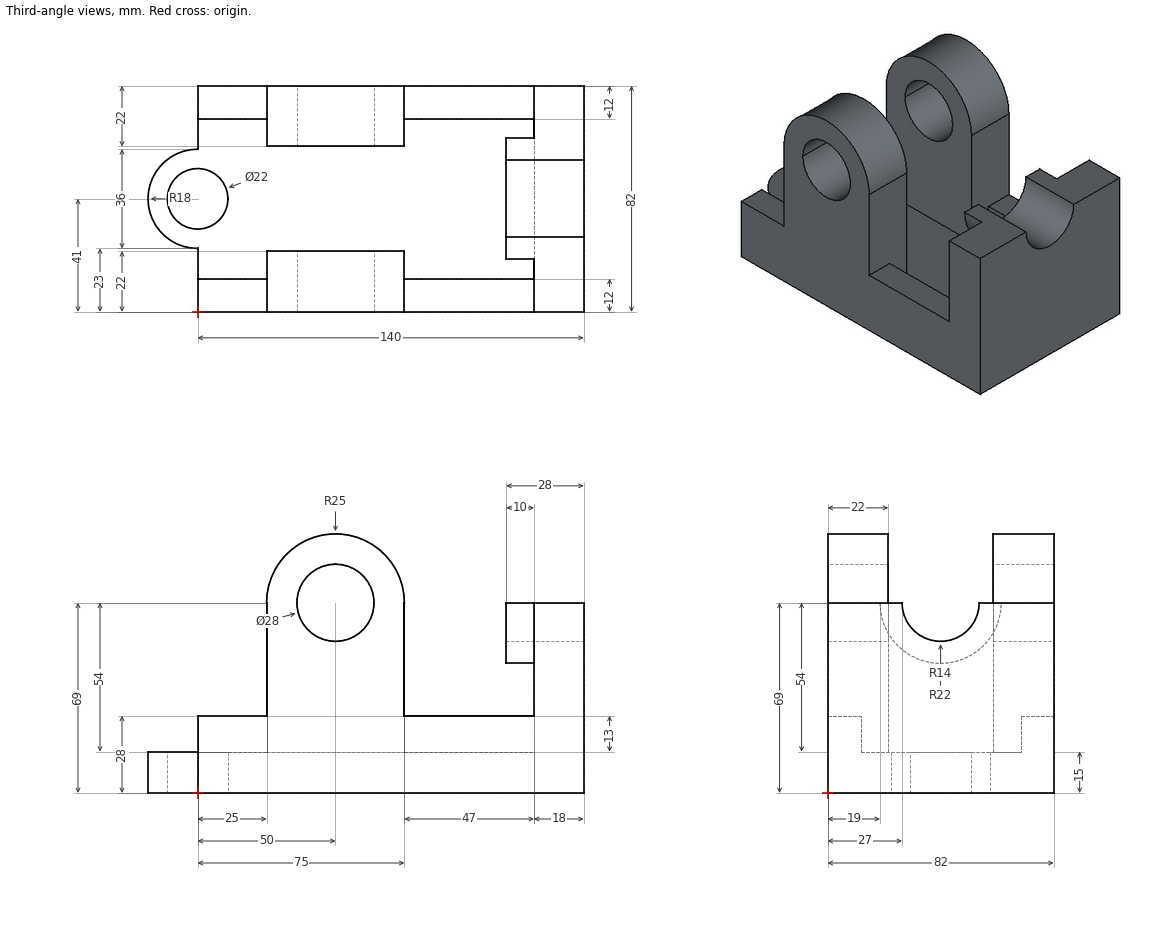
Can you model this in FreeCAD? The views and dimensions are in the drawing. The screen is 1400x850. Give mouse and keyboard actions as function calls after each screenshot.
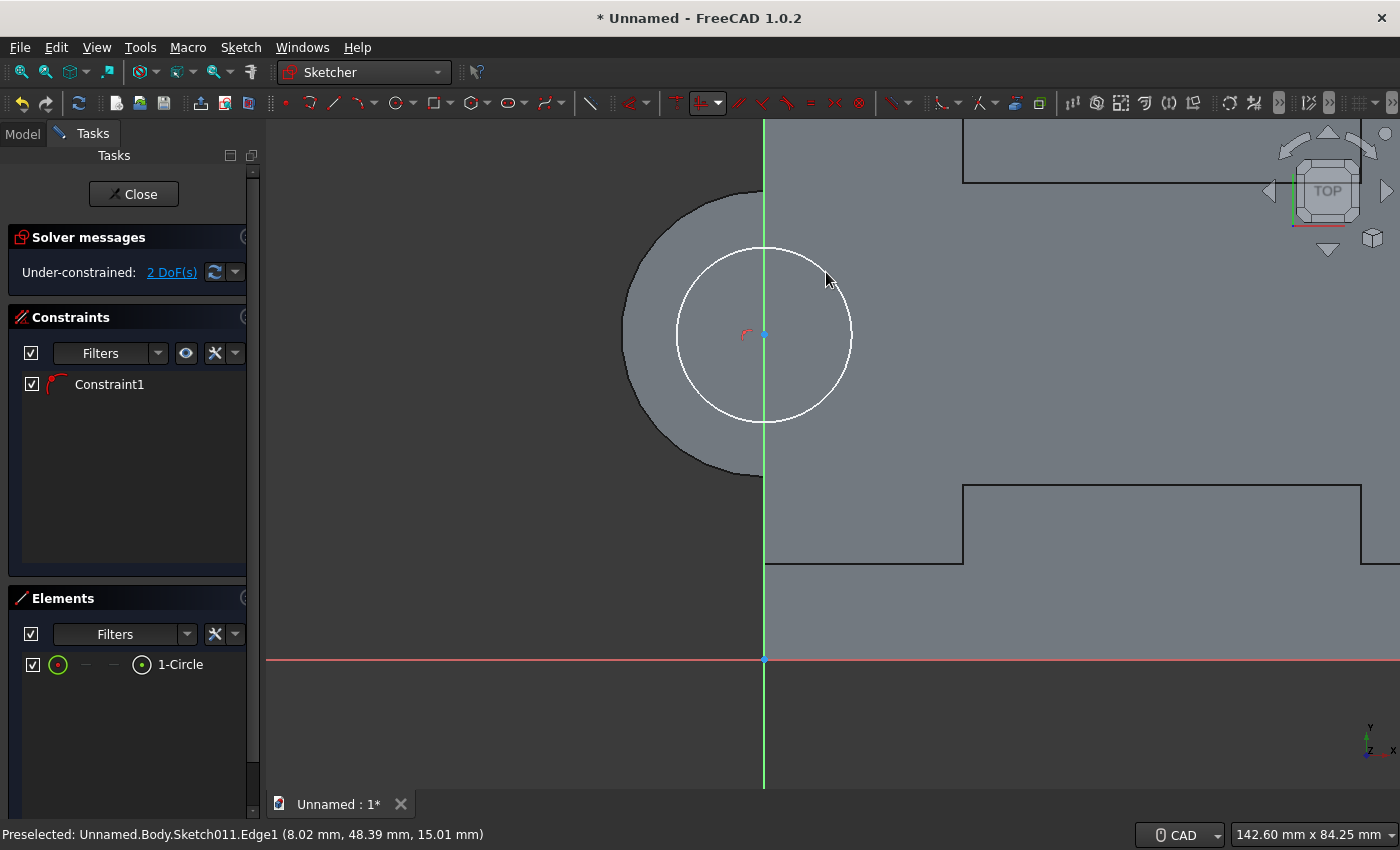
click(630, 104)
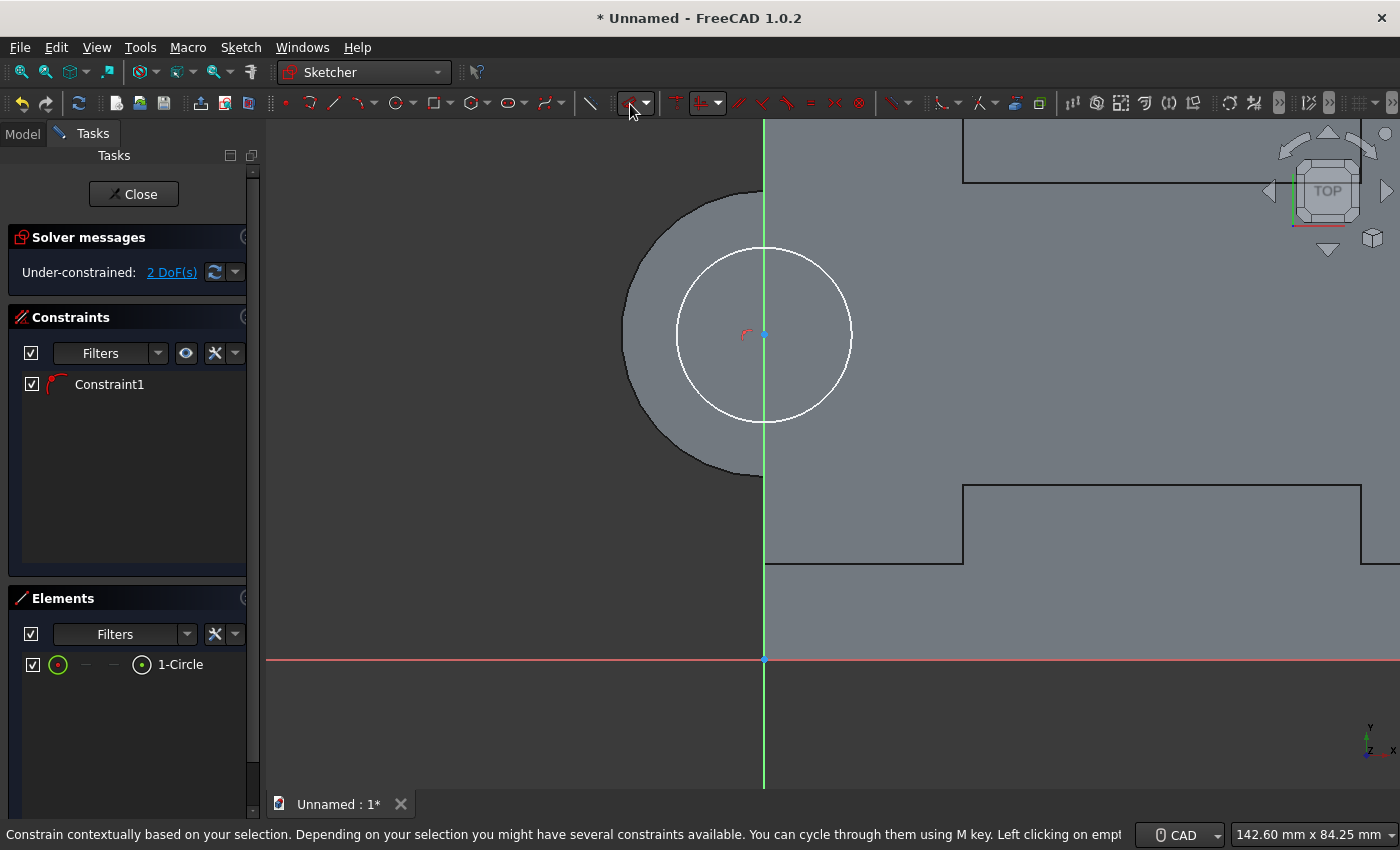
click(826, 273)
click(849, 250)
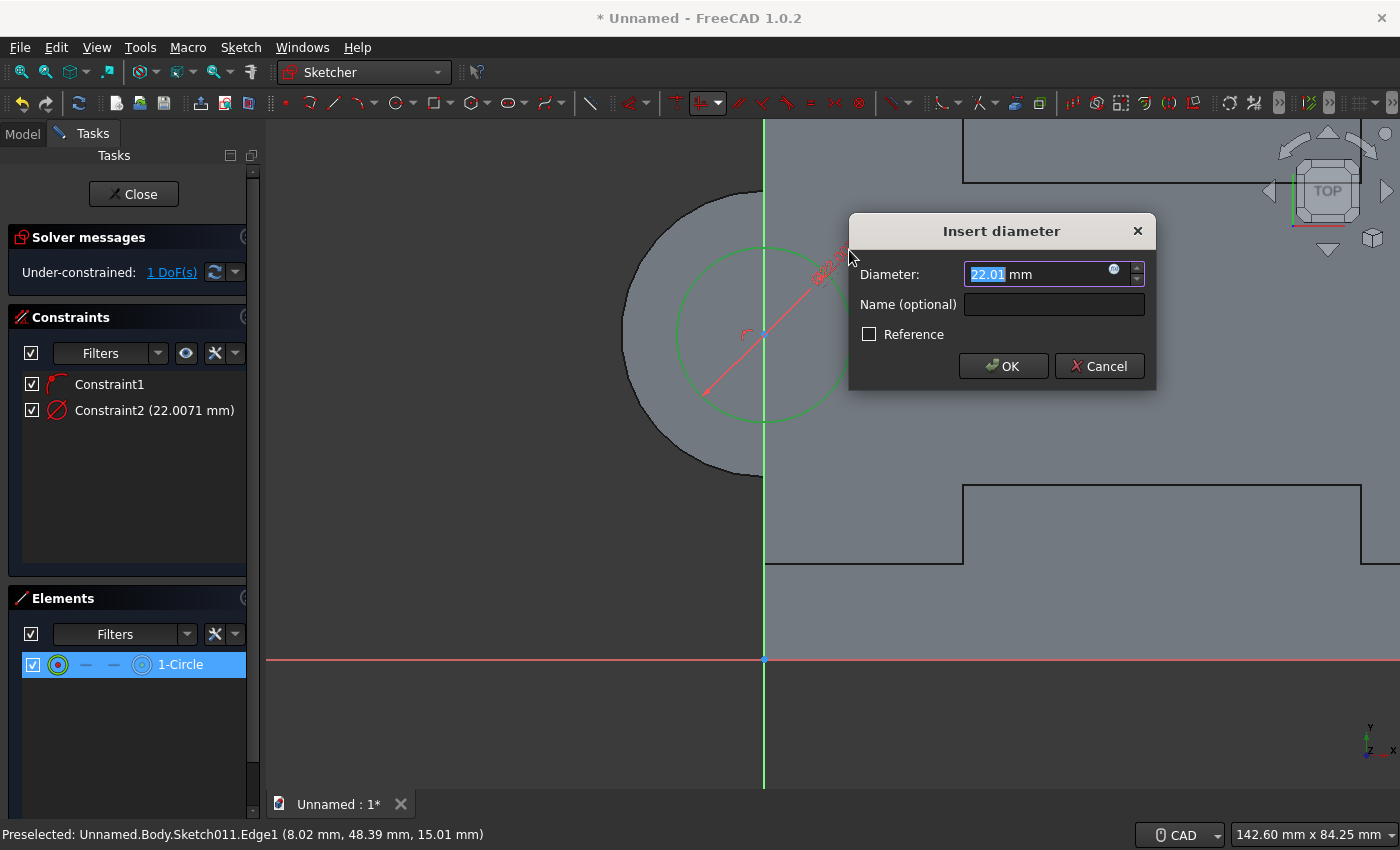
text(22)
key(Return)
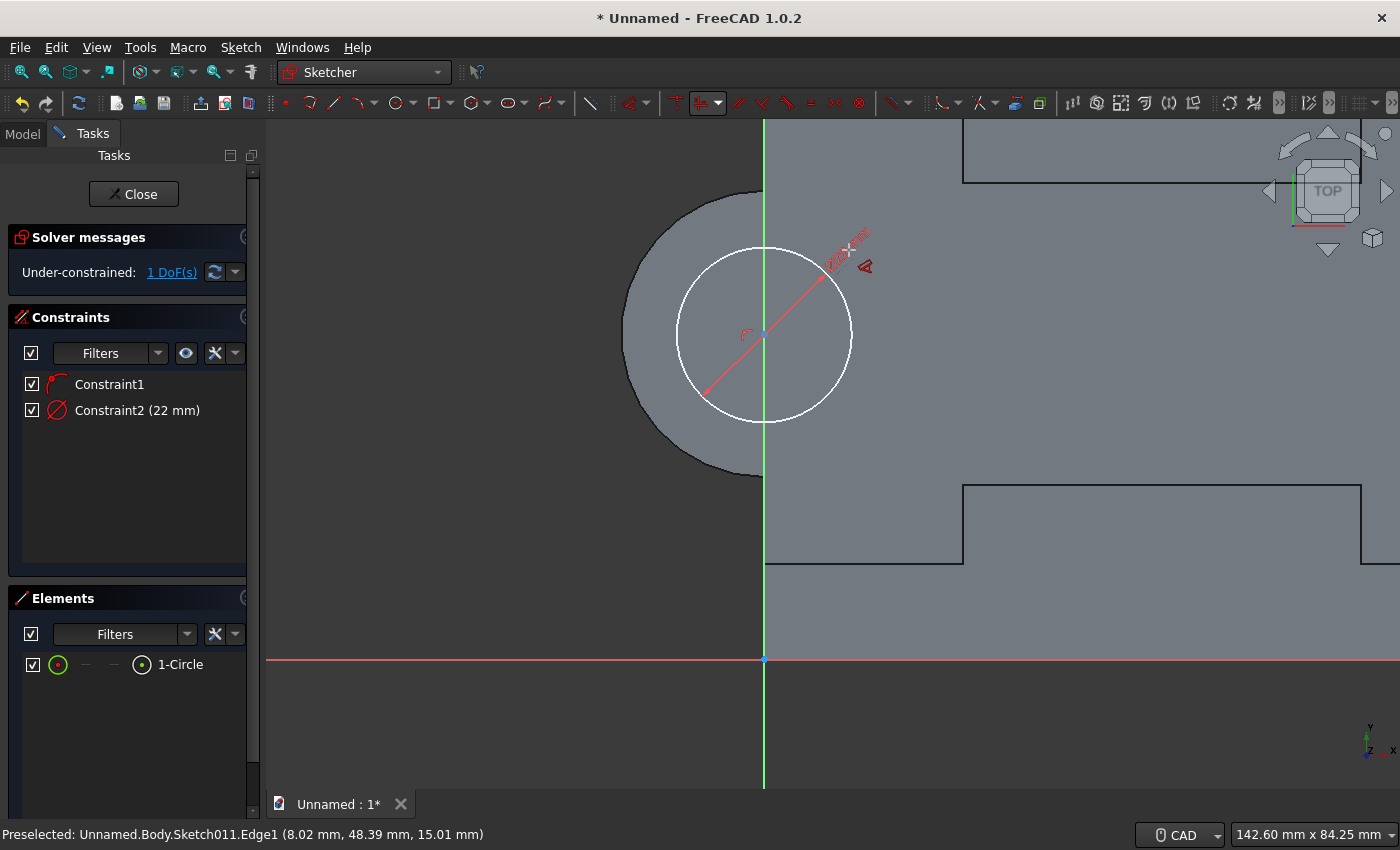
click(764, 335)
click(798, 497)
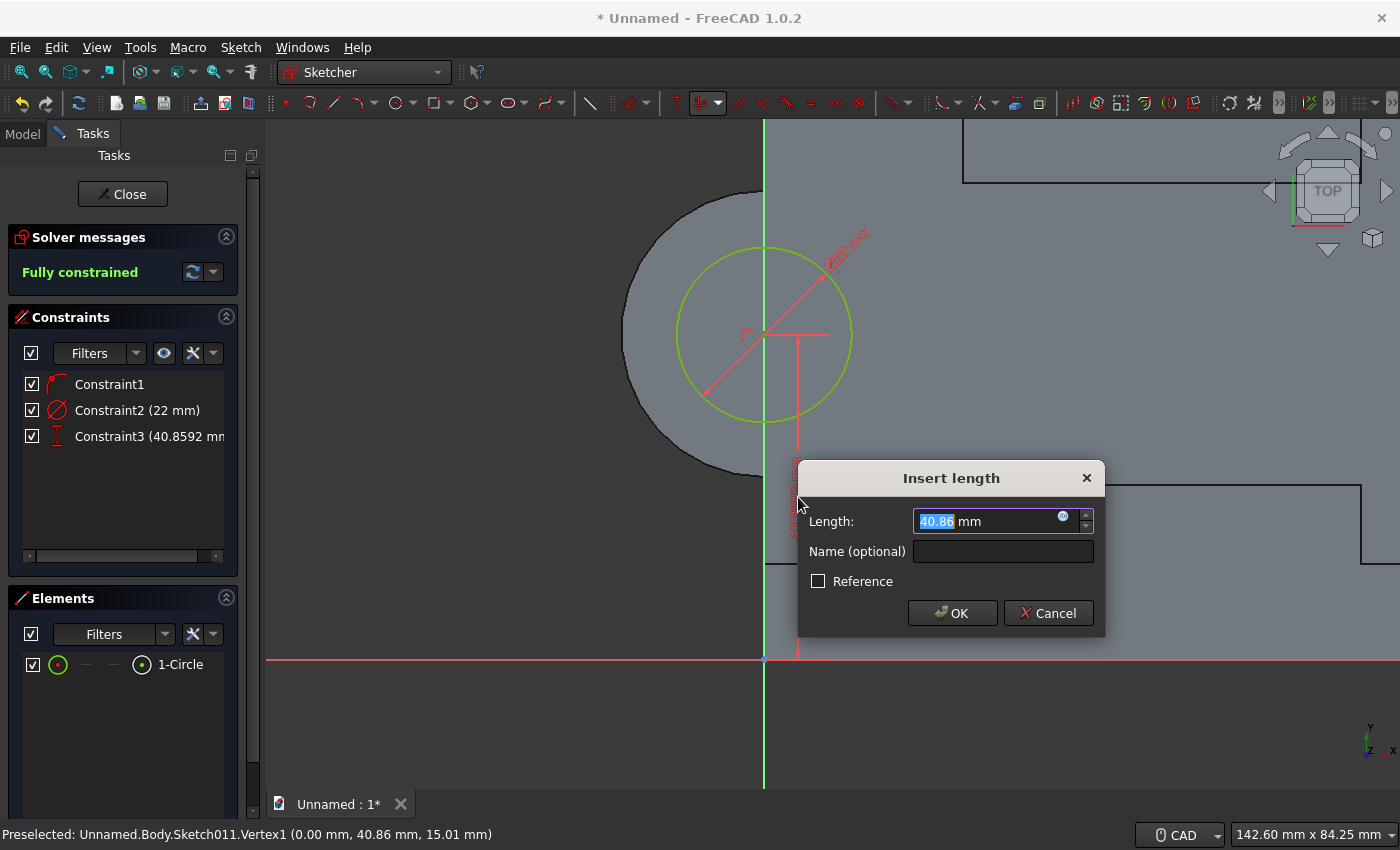
text(41)
key(Return)
key(Escape)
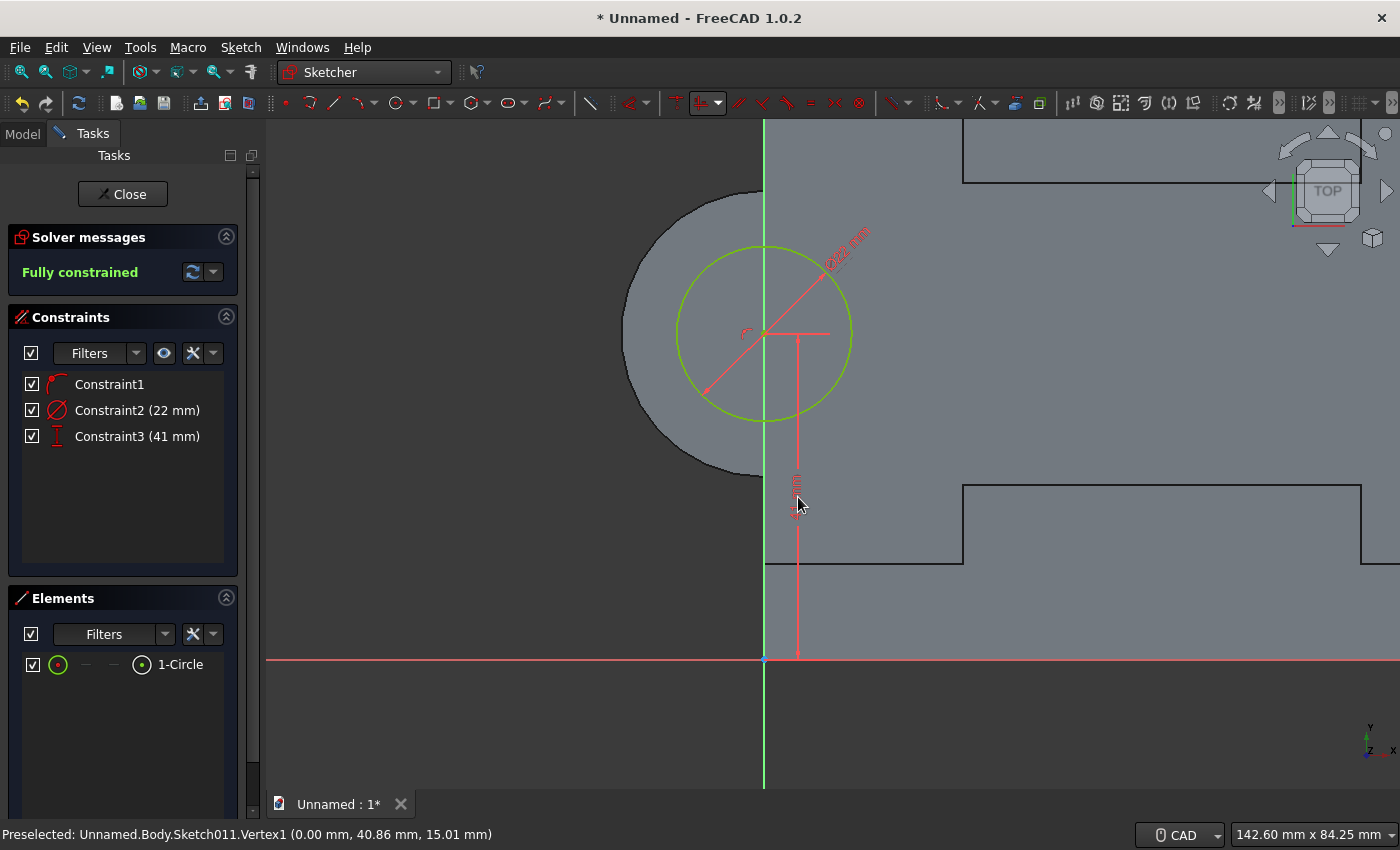
click(123, 194)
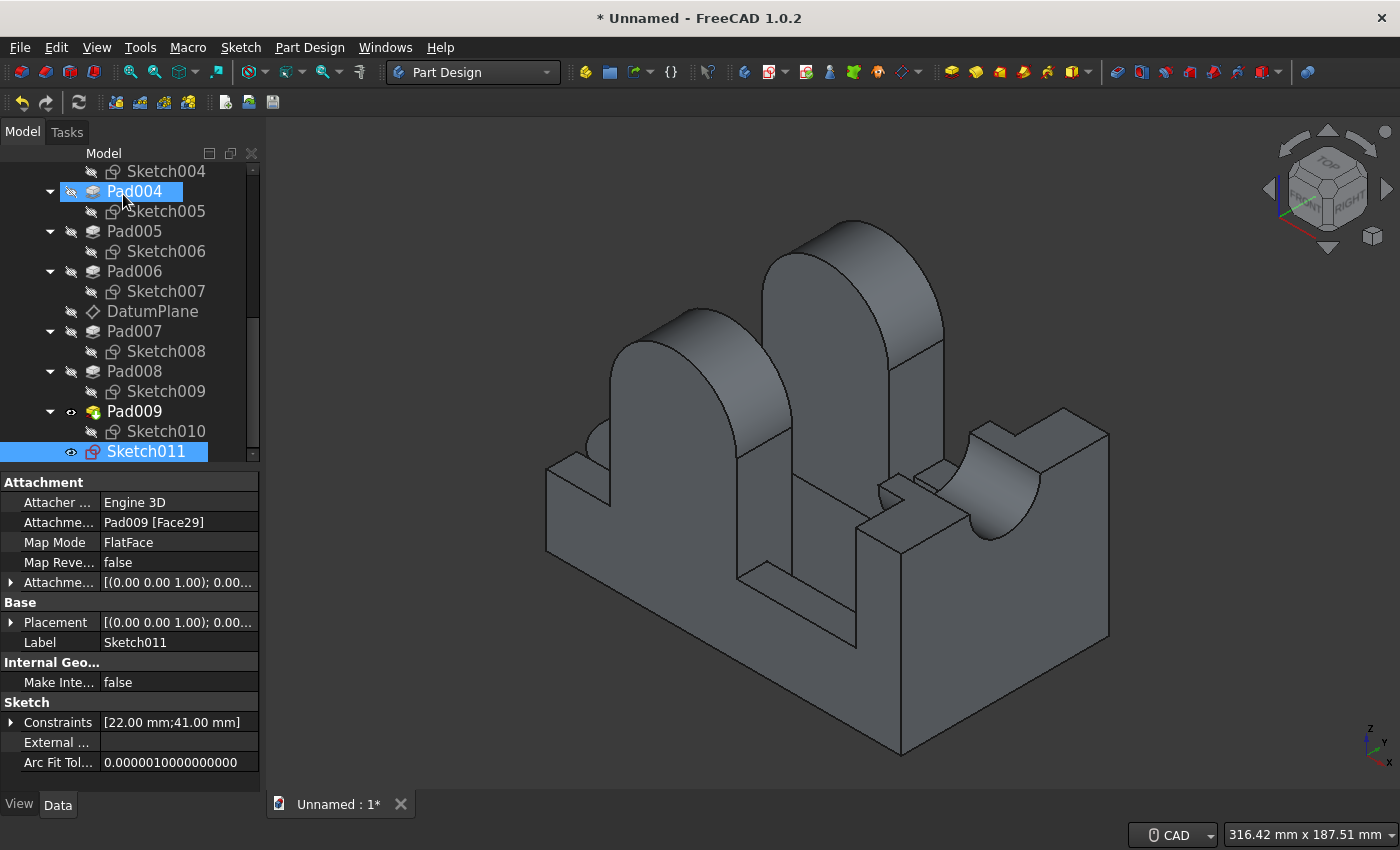
click(1118, 72)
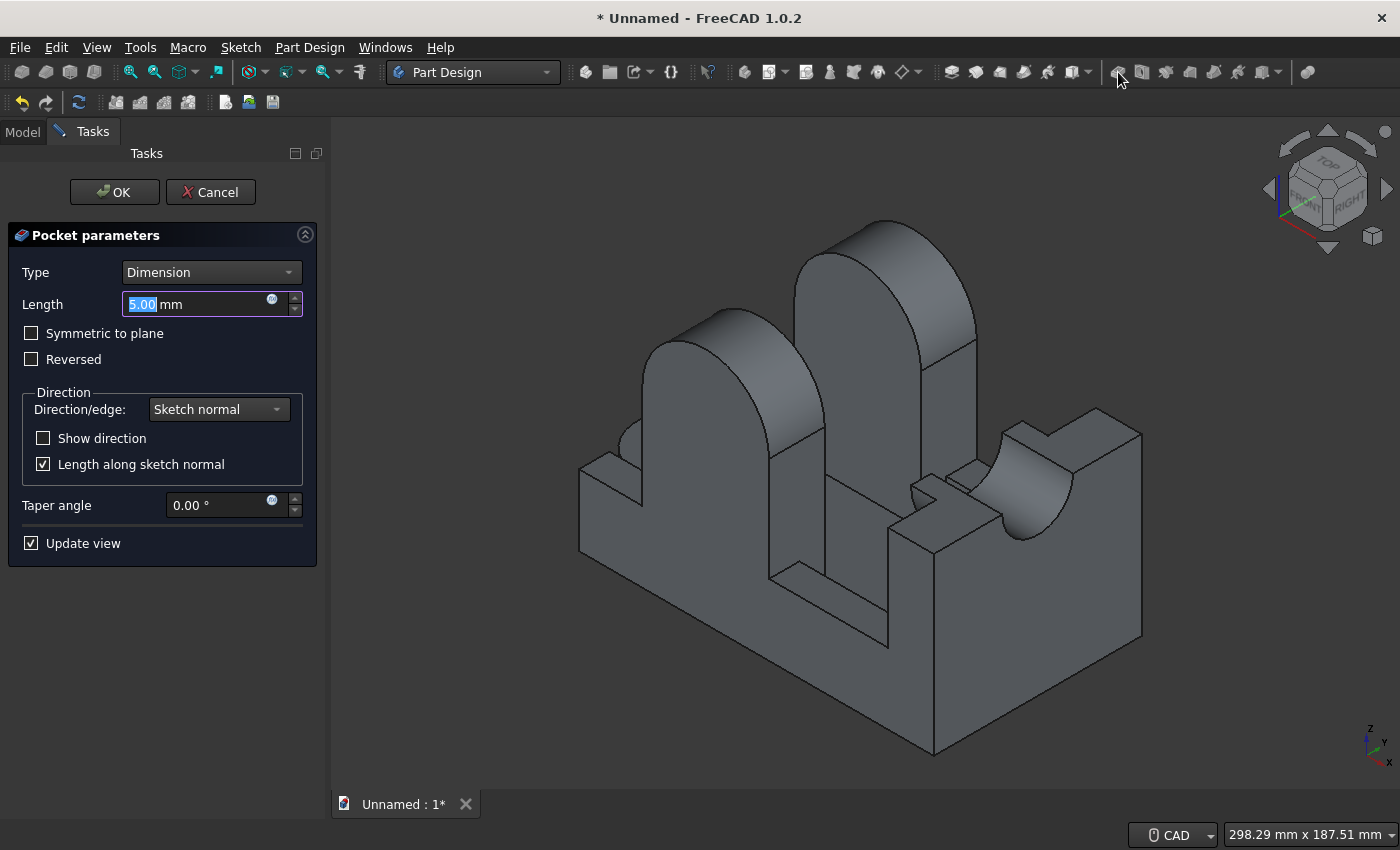
text(15)
key(Tab)